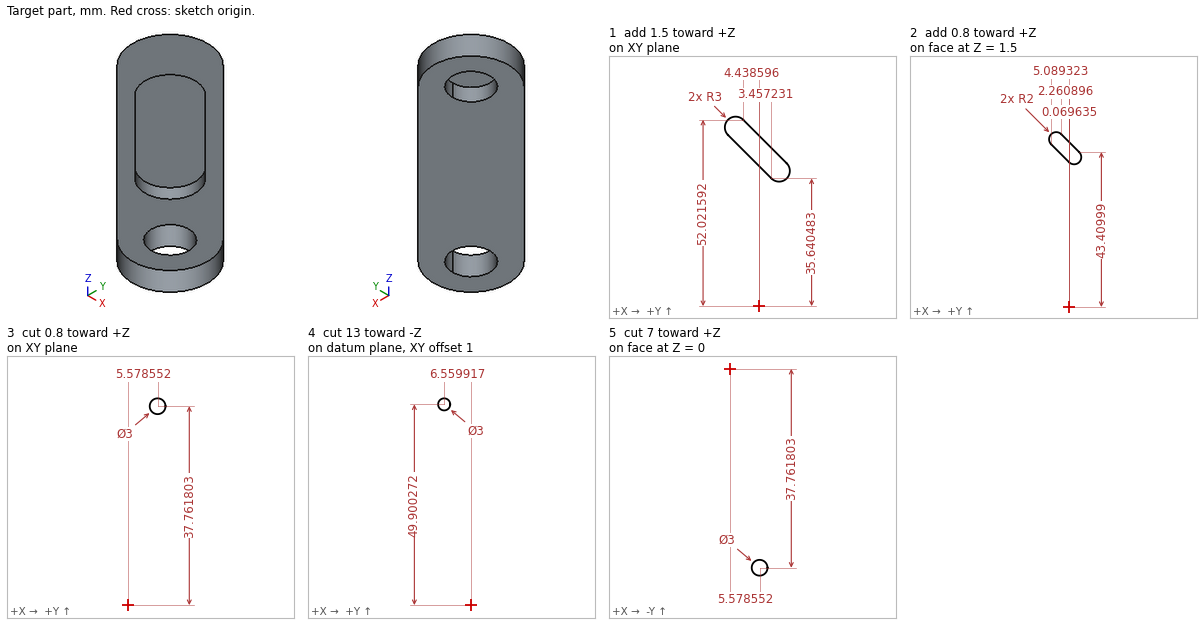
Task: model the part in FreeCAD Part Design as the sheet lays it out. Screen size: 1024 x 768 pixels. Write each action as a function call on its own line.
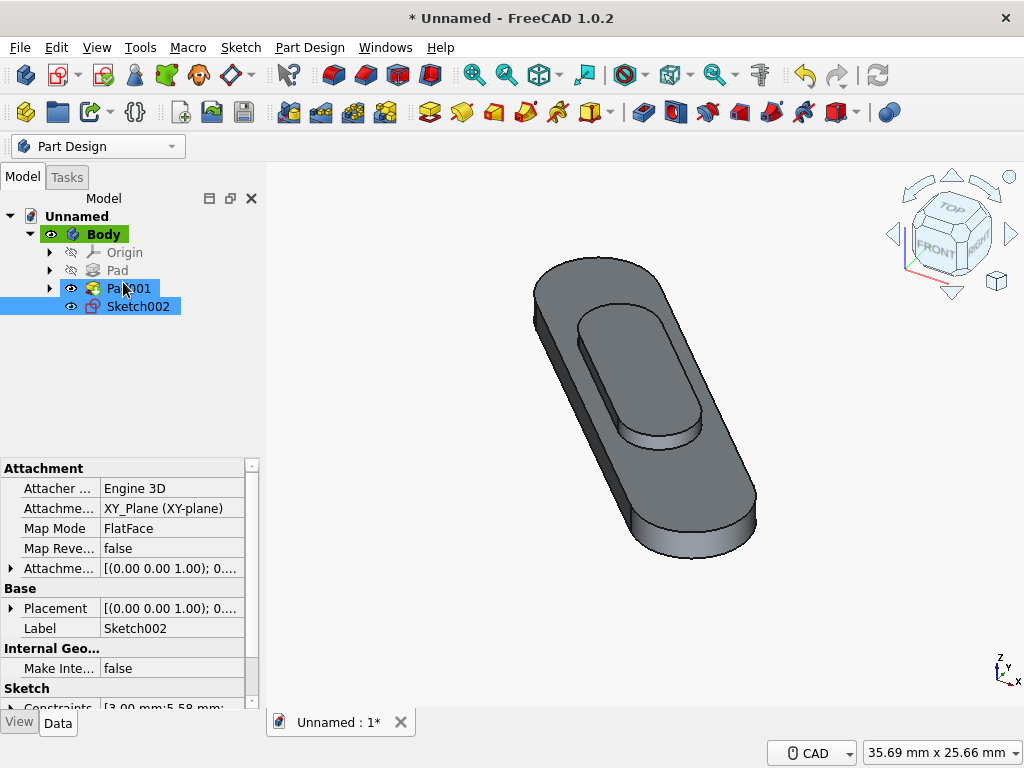
click(644, 112)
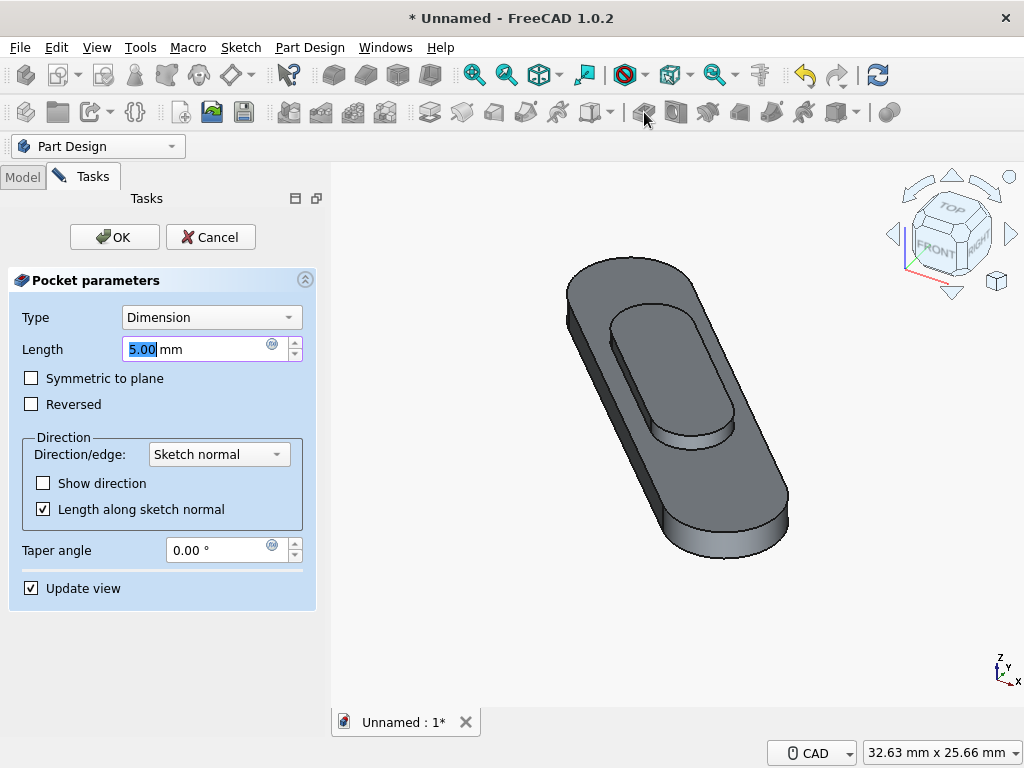
text(0.8)
key(Tab)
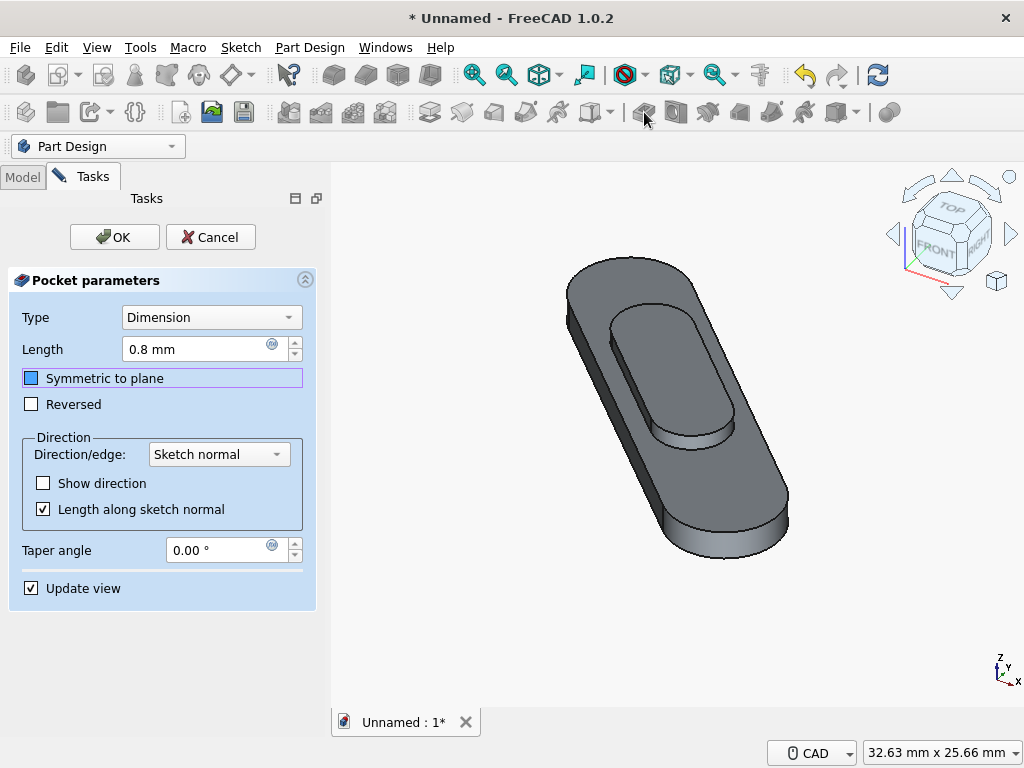
click(30, 404)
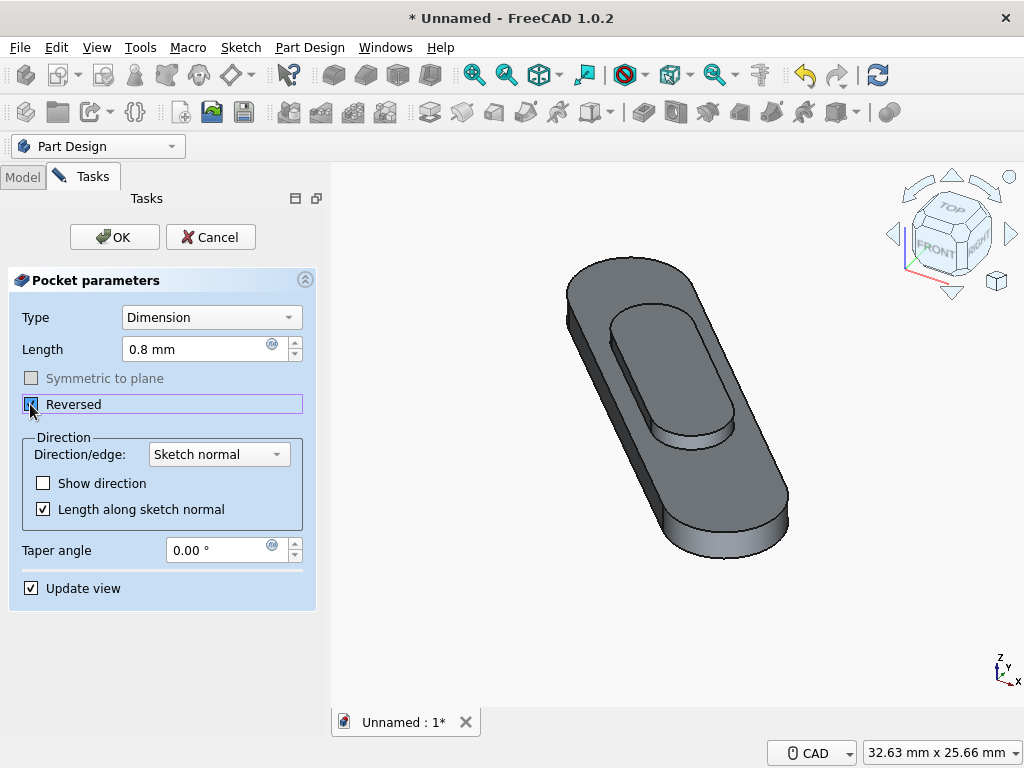
click(115, 237)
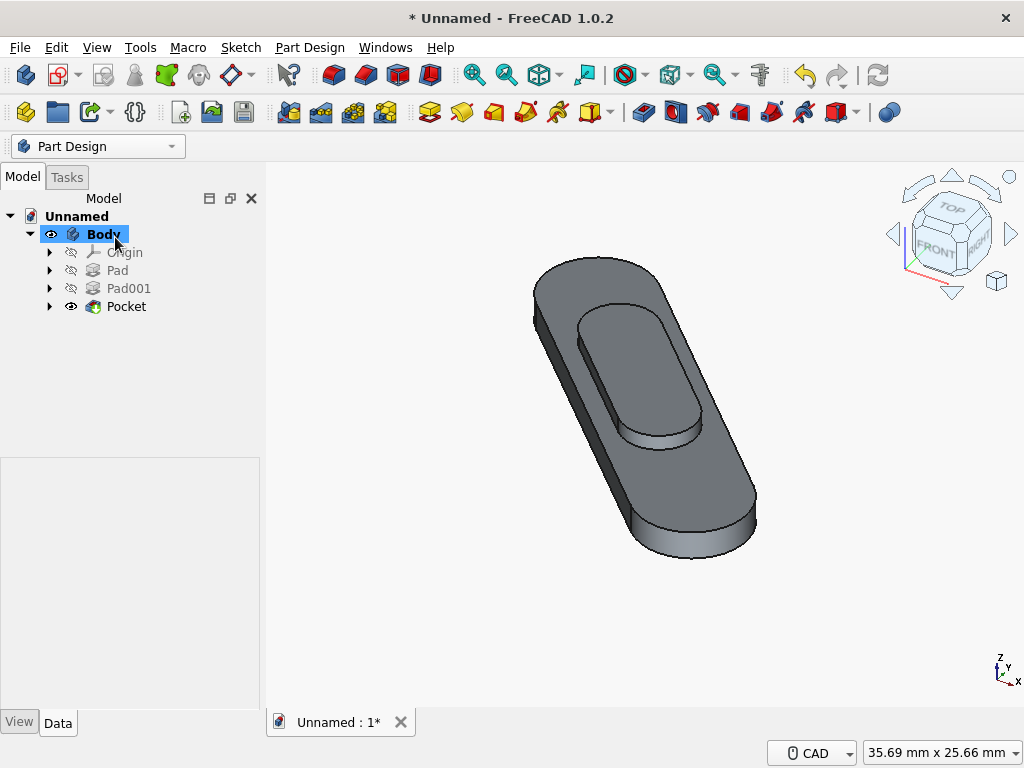
click(50, 252)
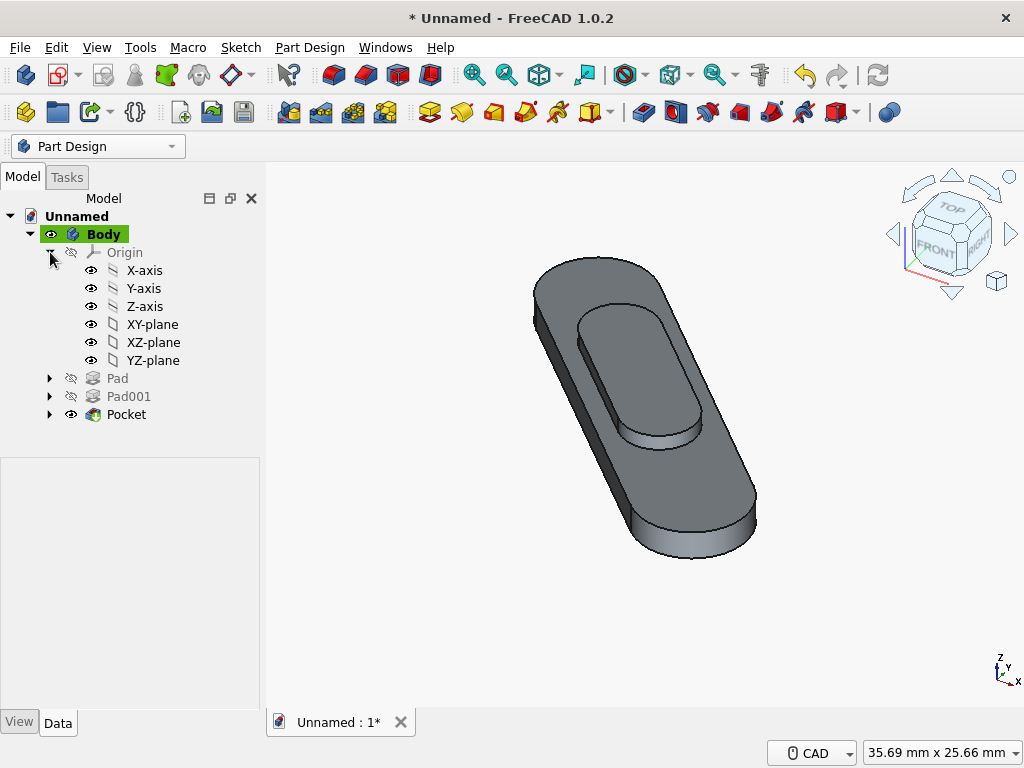
click(136, 324)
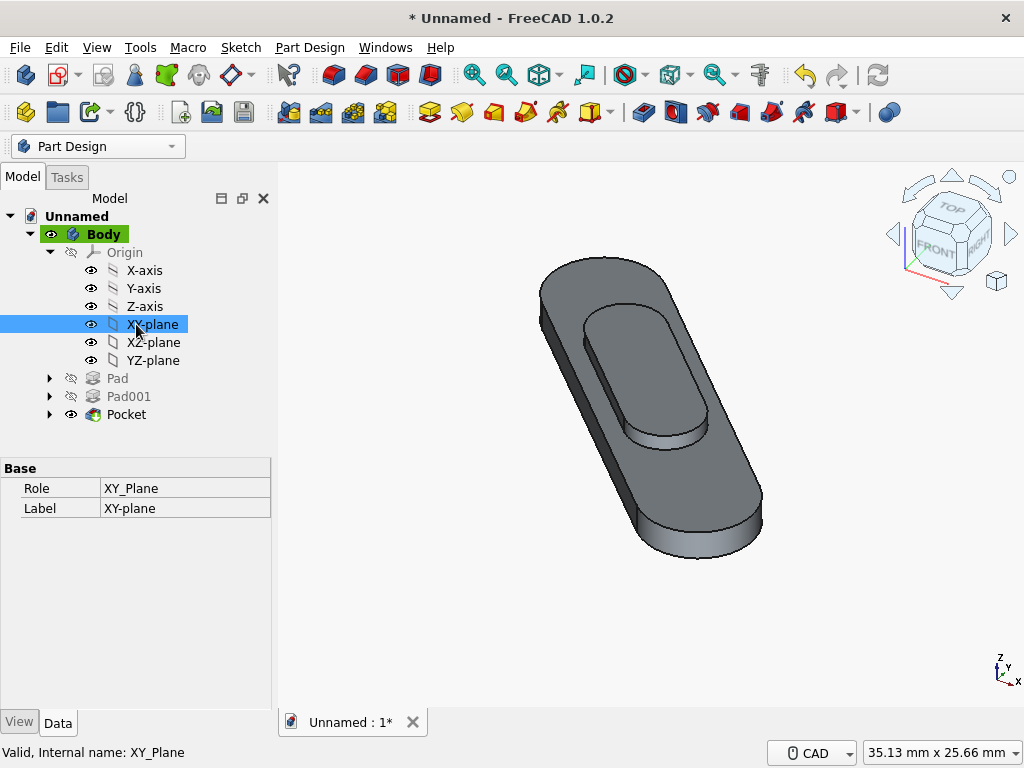
click(232, 76)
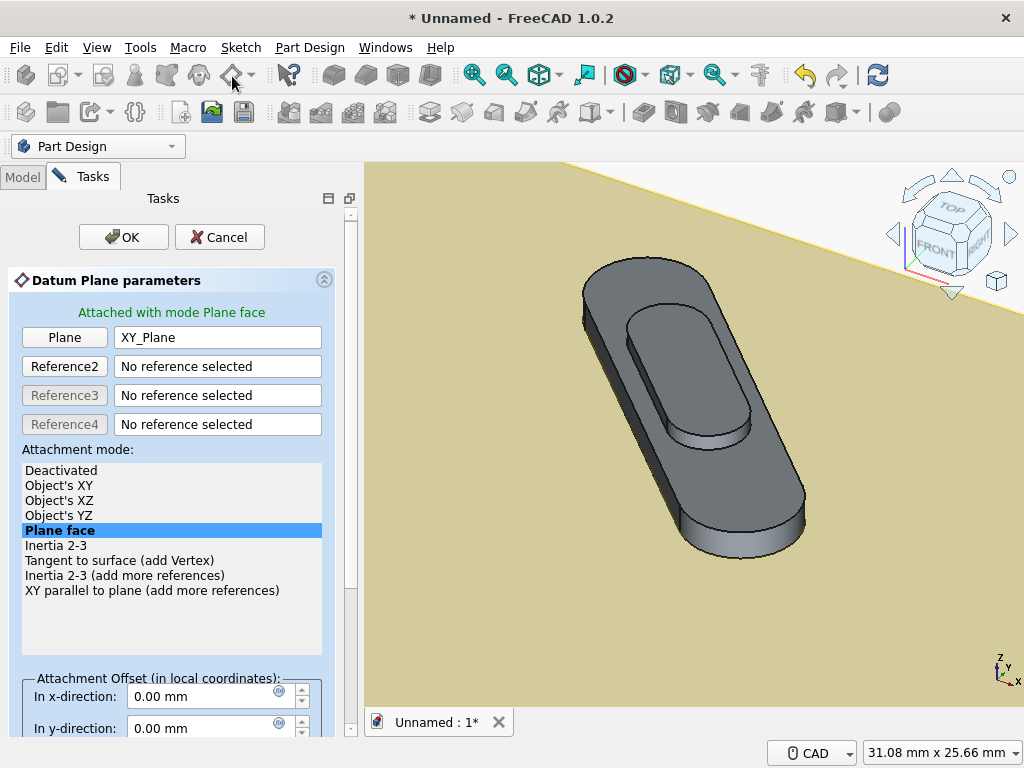
scroll(351, 472, down, 2)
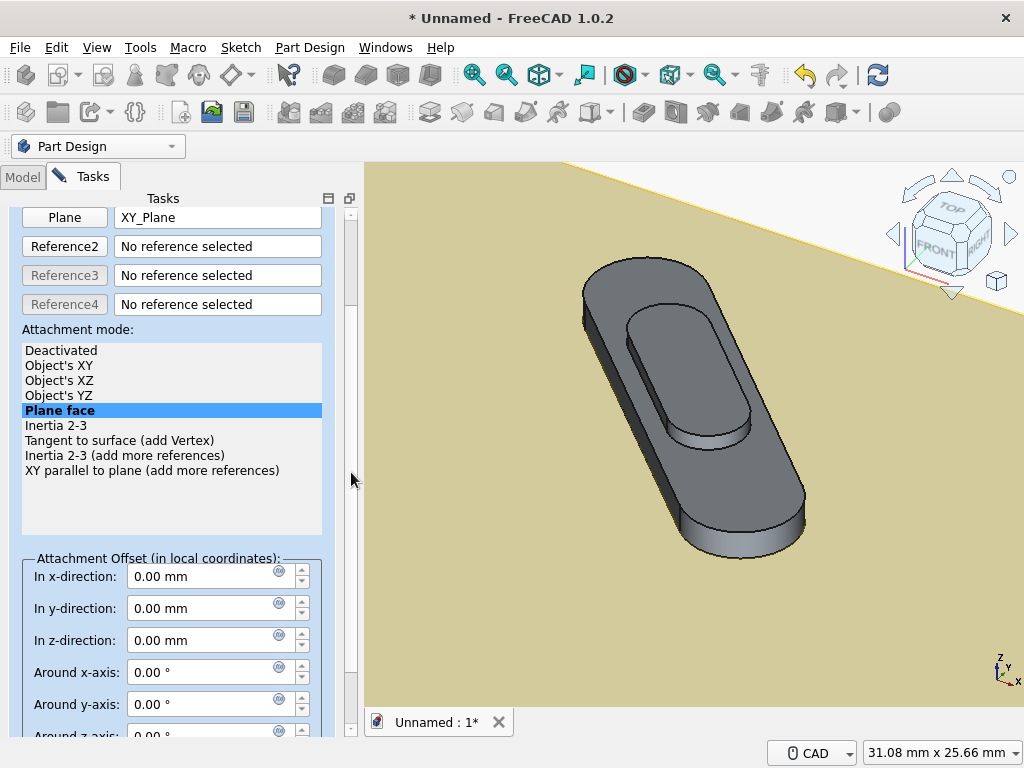
triple_click(210, 640)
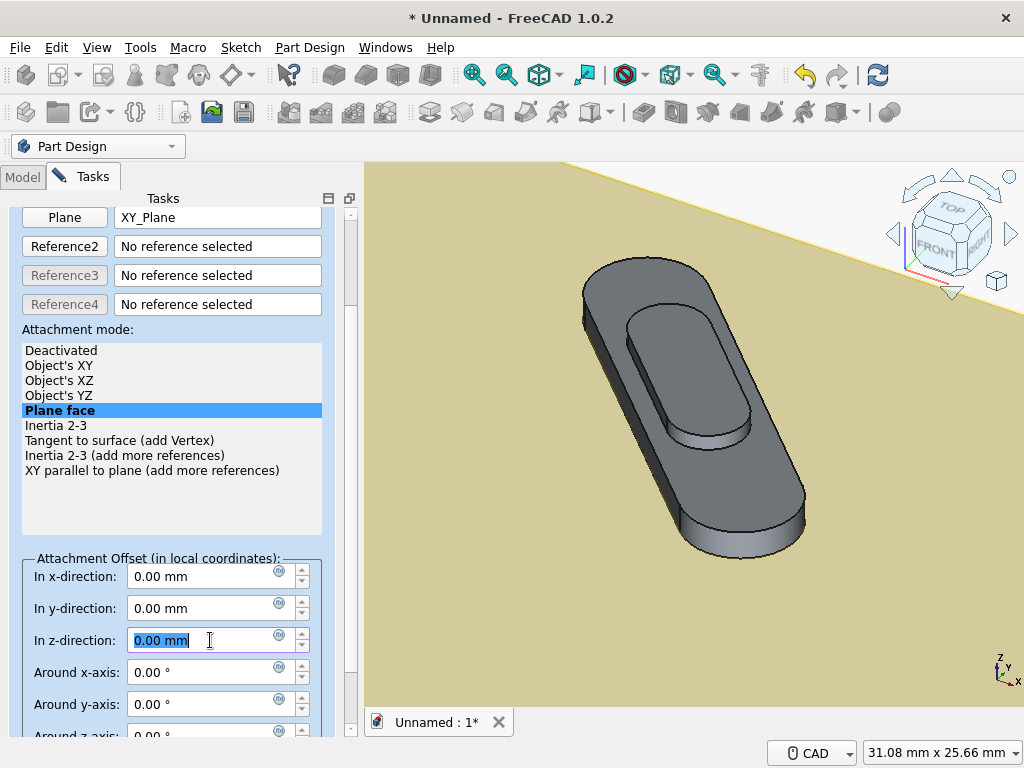
text(1)
key(Tab)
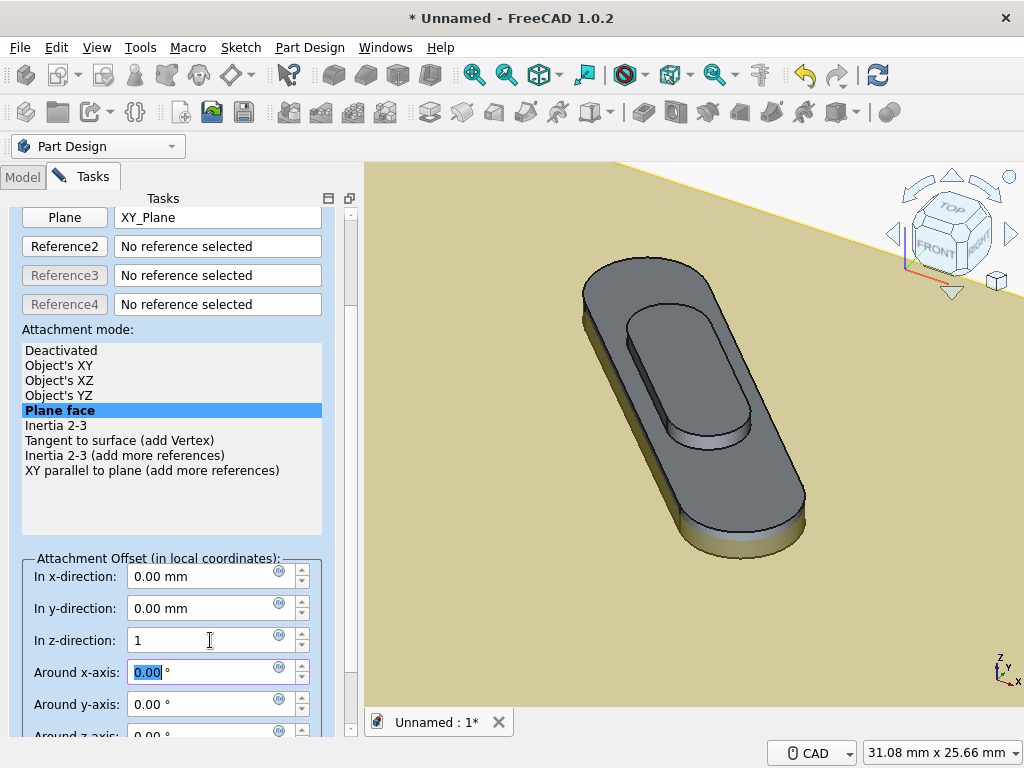
scroll(351, 472, up, 3)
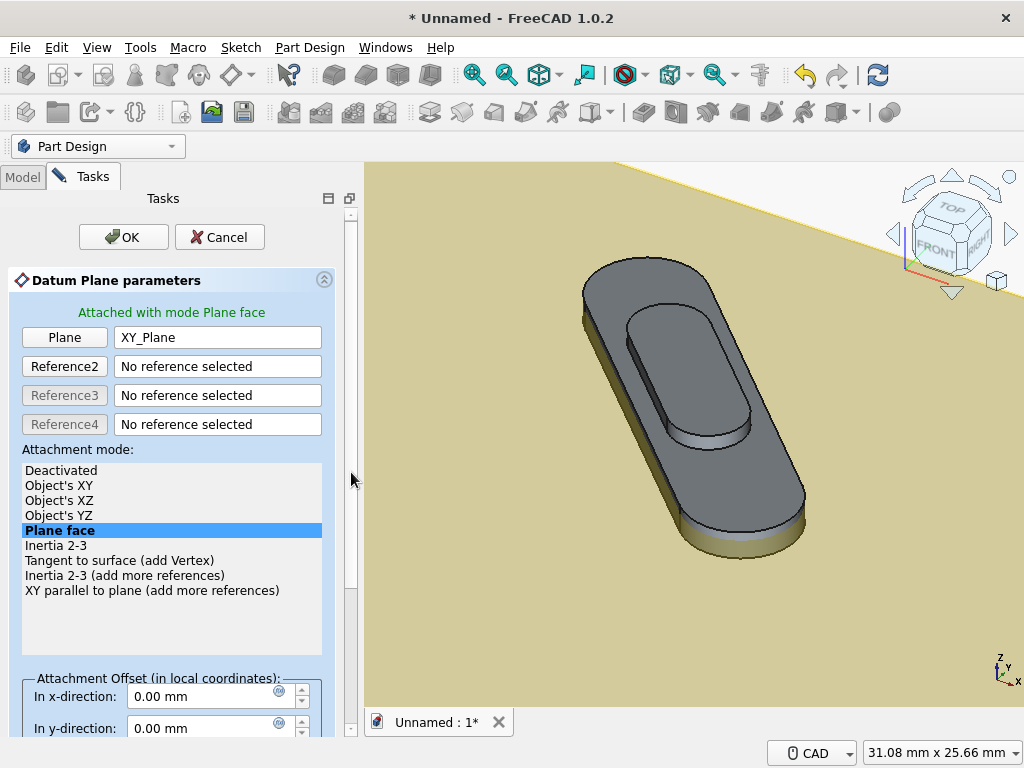
click(124, 237)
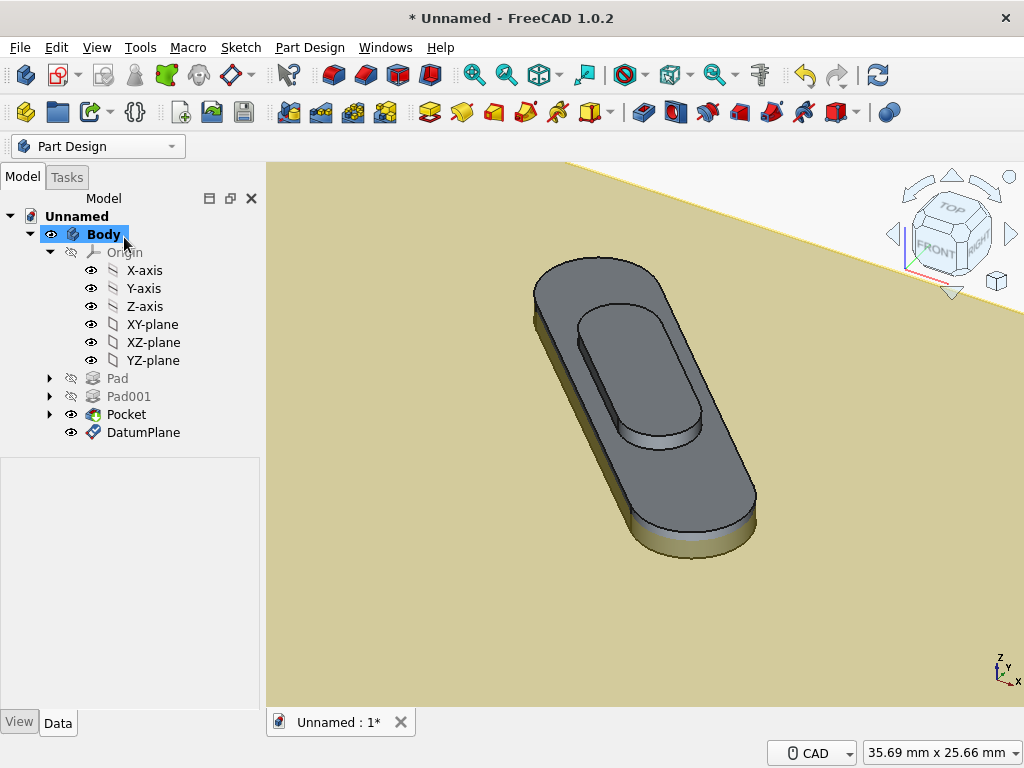
click(116, 432)